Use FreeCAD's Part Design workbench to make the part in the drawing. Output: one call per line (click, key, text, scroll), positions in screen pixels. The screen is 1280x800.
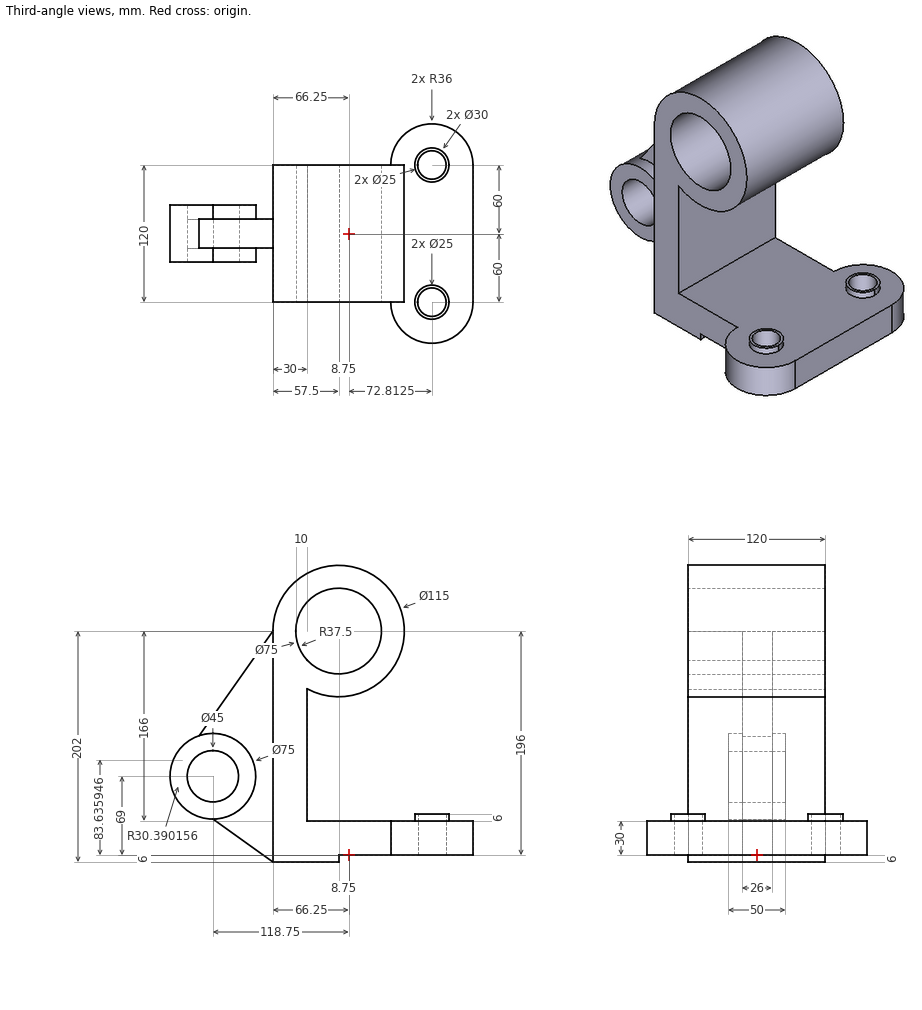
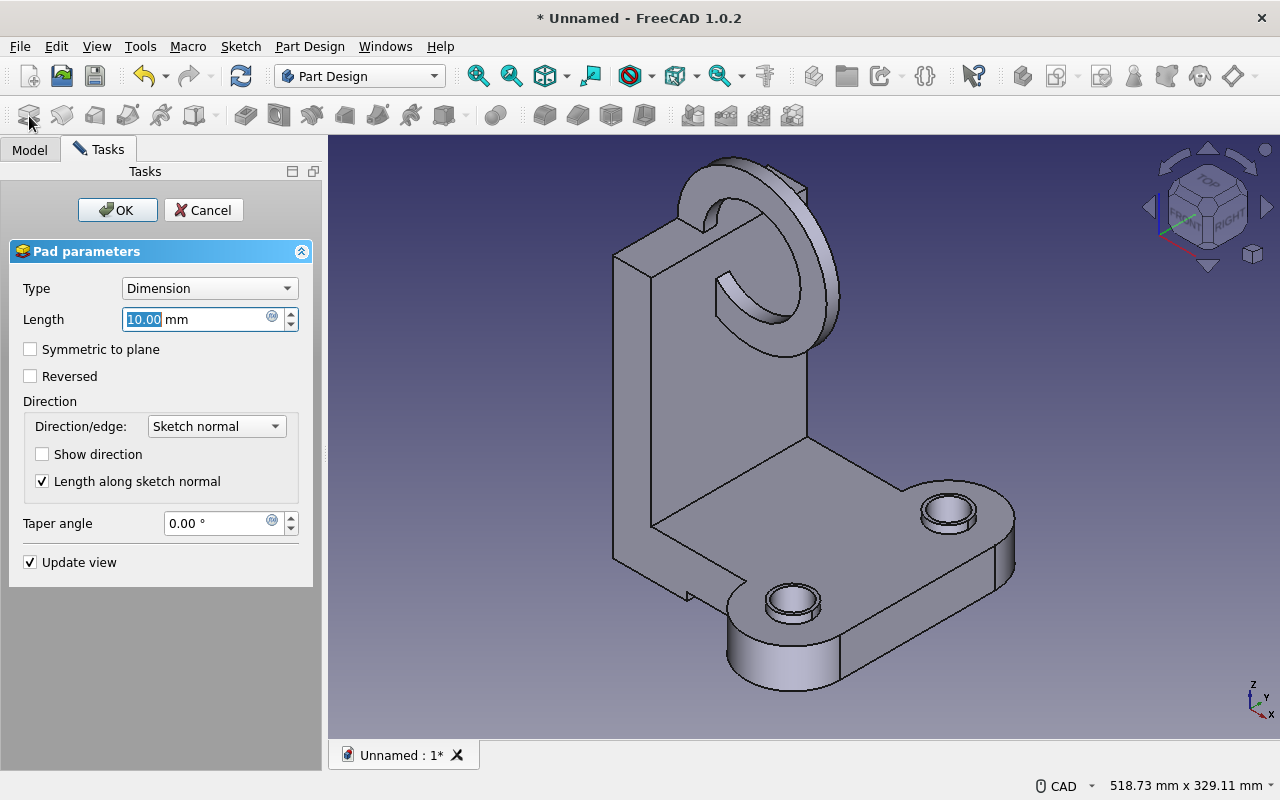
text(120)
key(Tab)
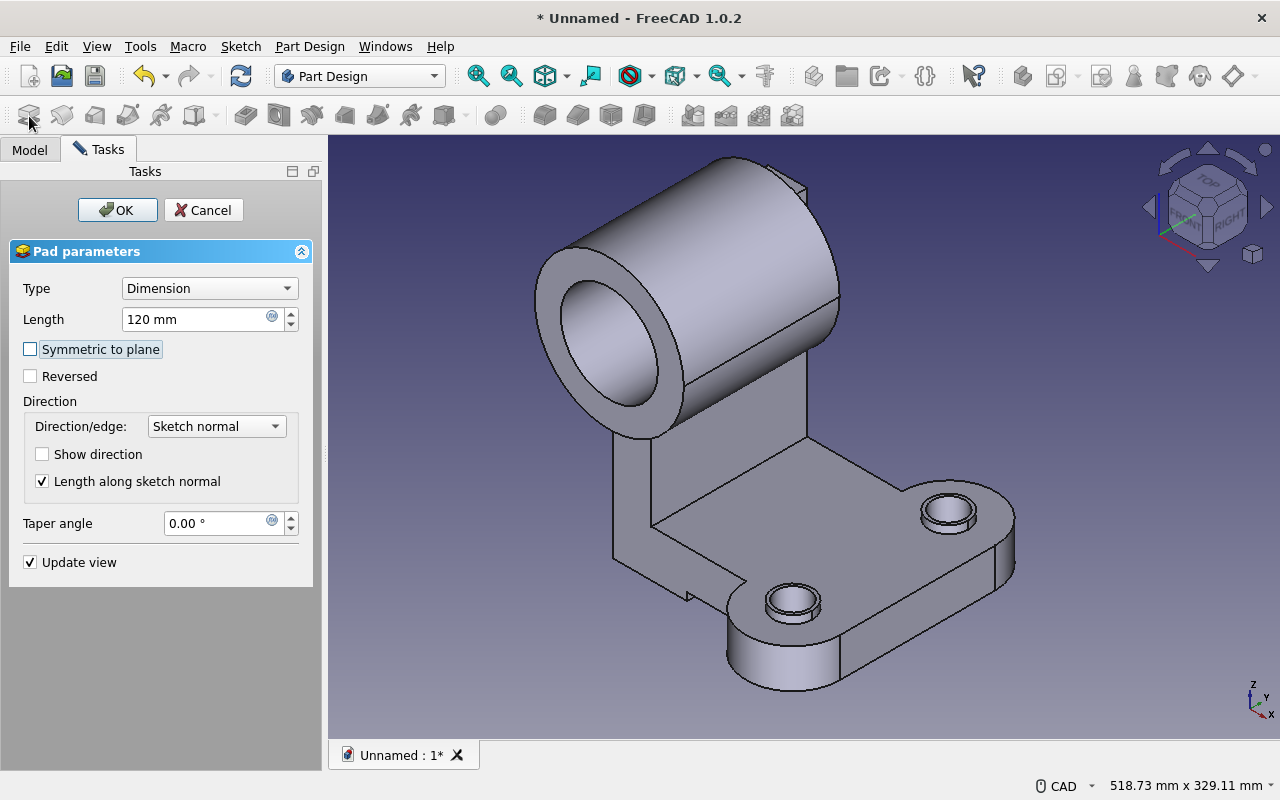
click(31, 349)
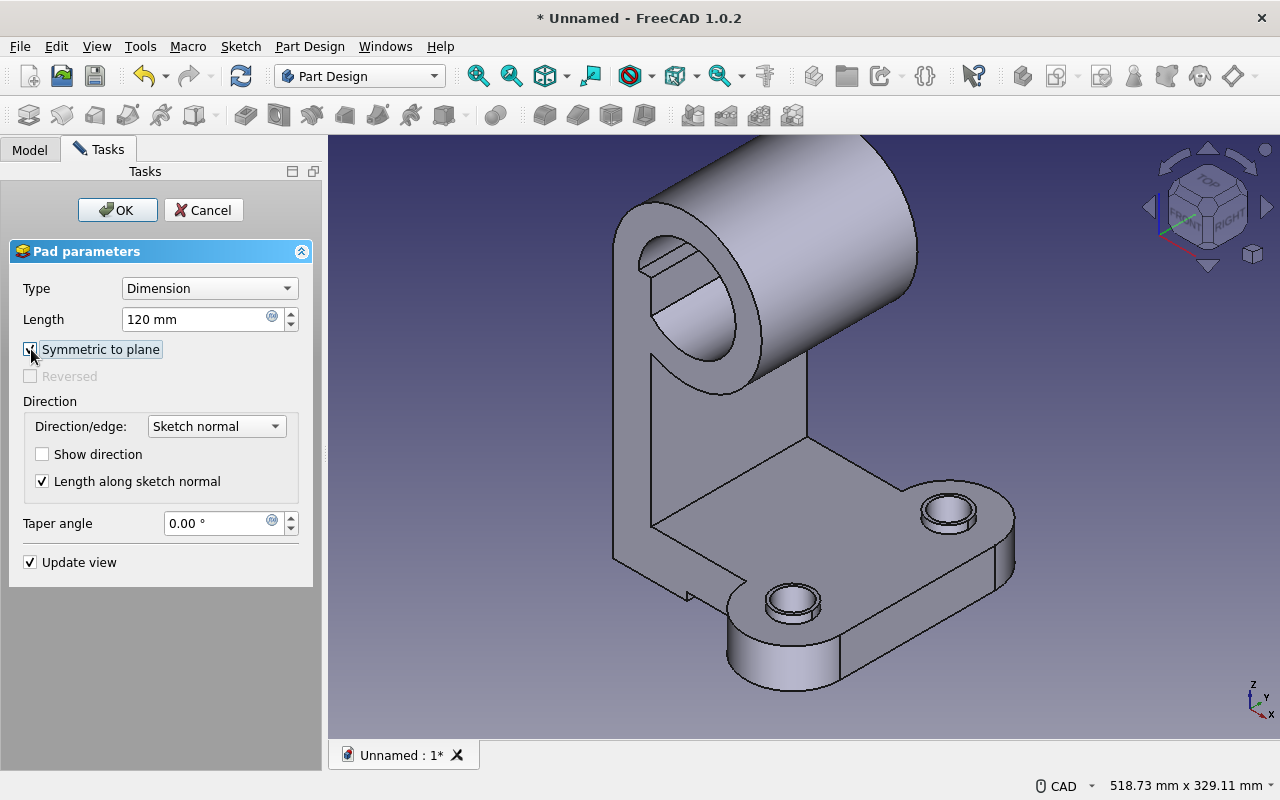
click(118, 210)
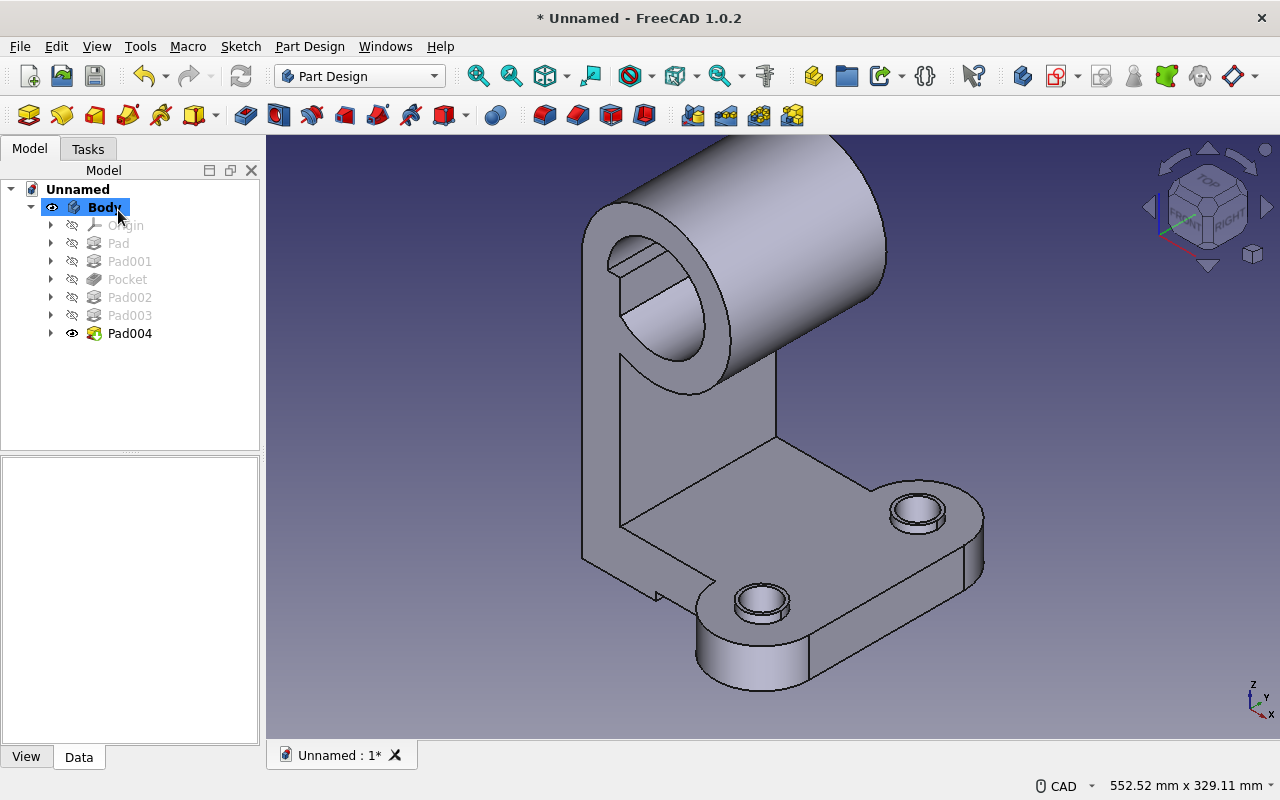
key(v)
key(f)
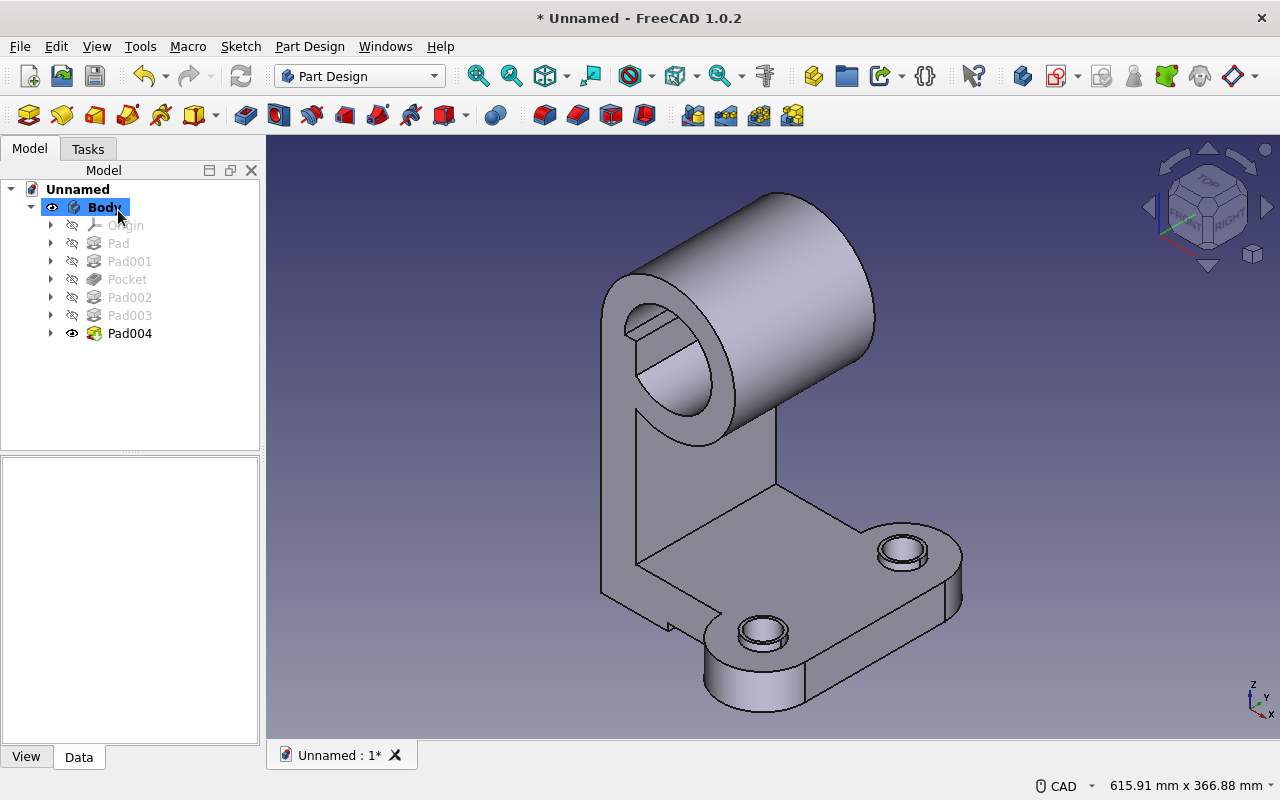
key(4)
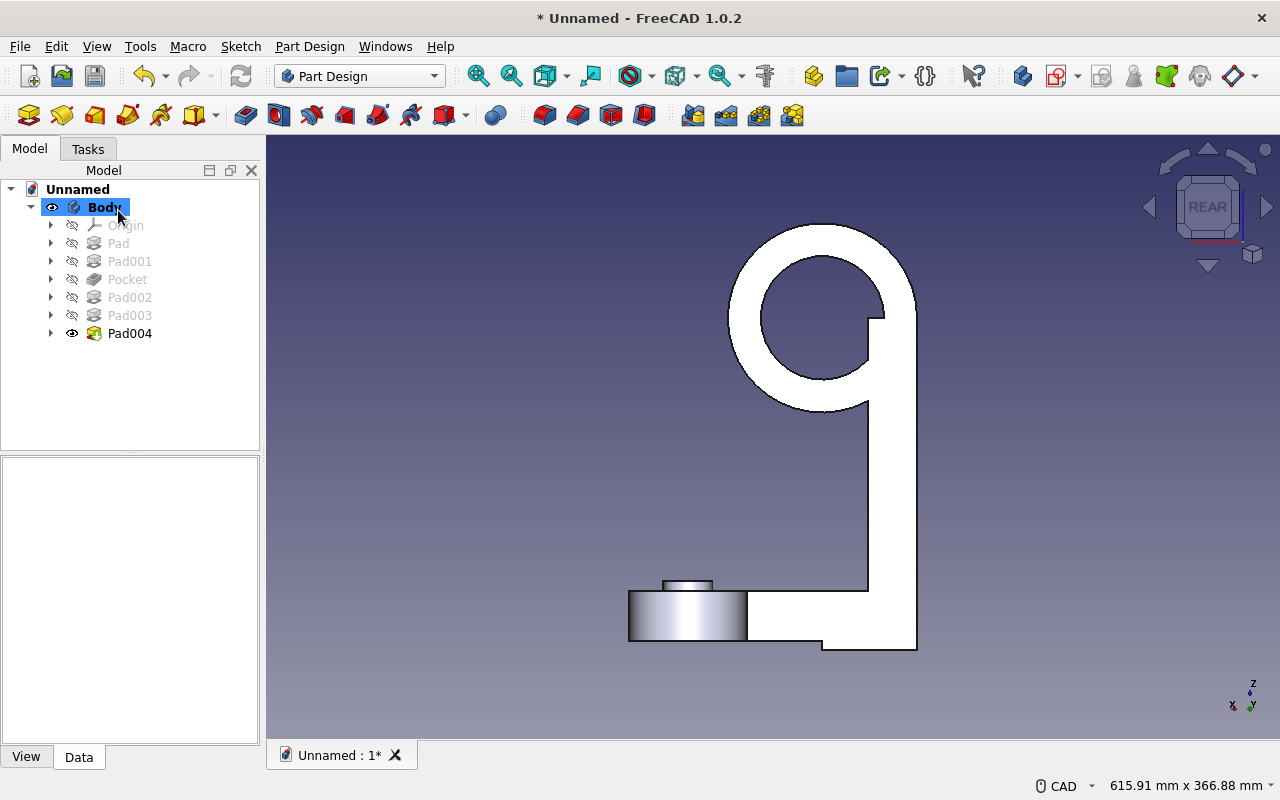
click(877, 619)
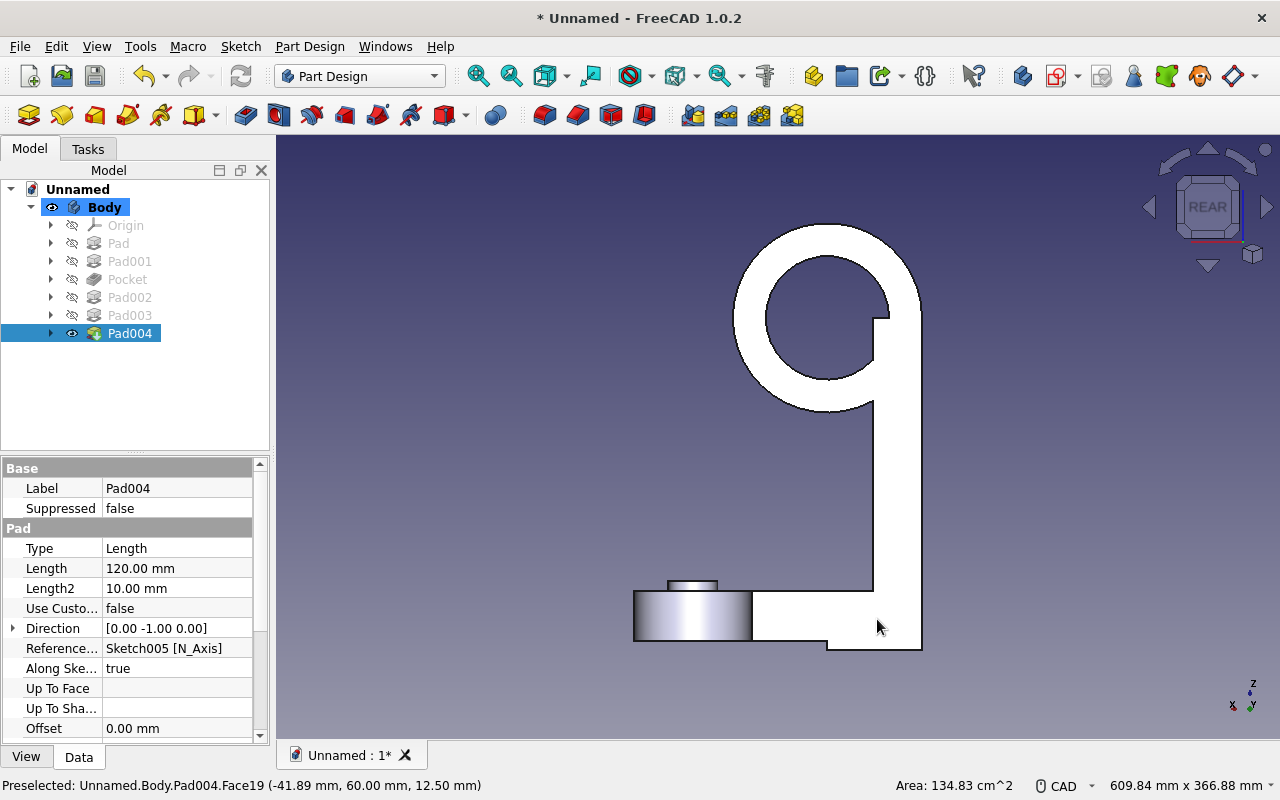
click(1056, 76)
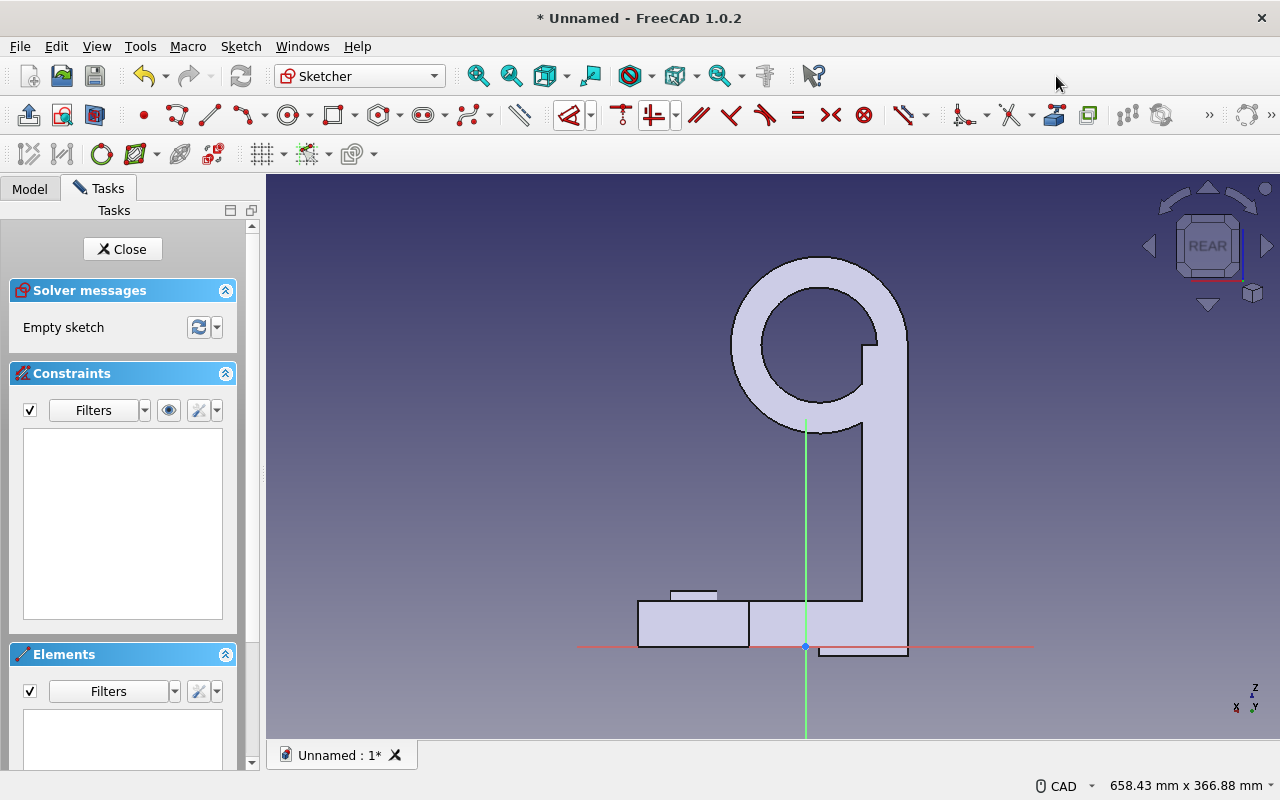
key(q)
key(s)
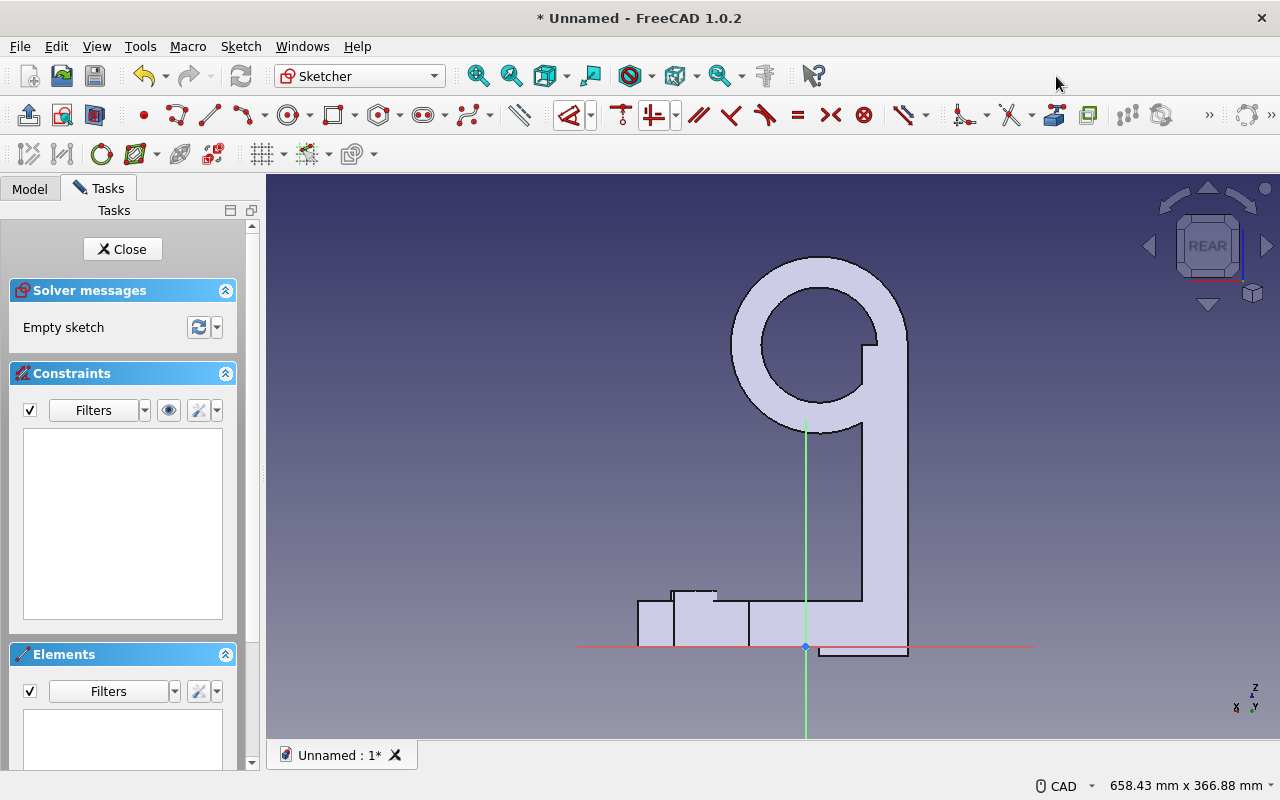
scroll(890, 353, up, 11)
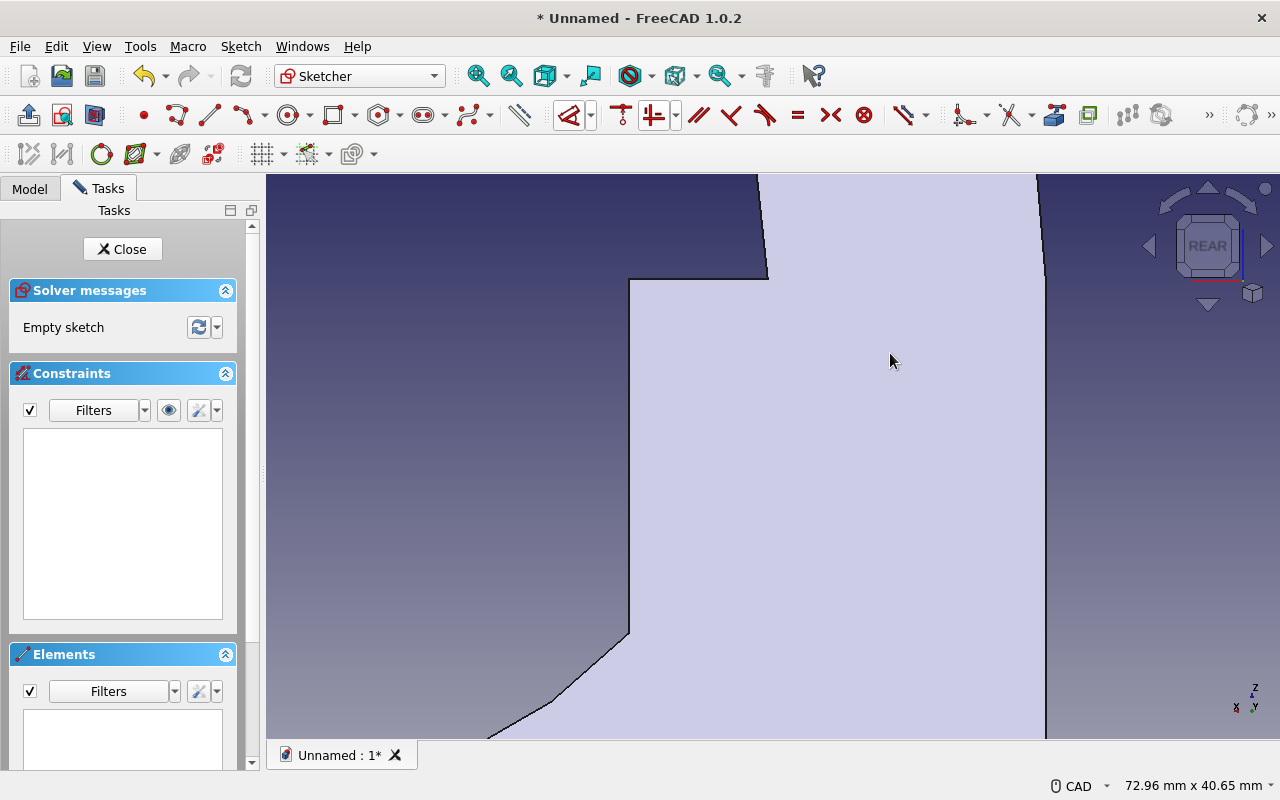
key(g)
key(m)